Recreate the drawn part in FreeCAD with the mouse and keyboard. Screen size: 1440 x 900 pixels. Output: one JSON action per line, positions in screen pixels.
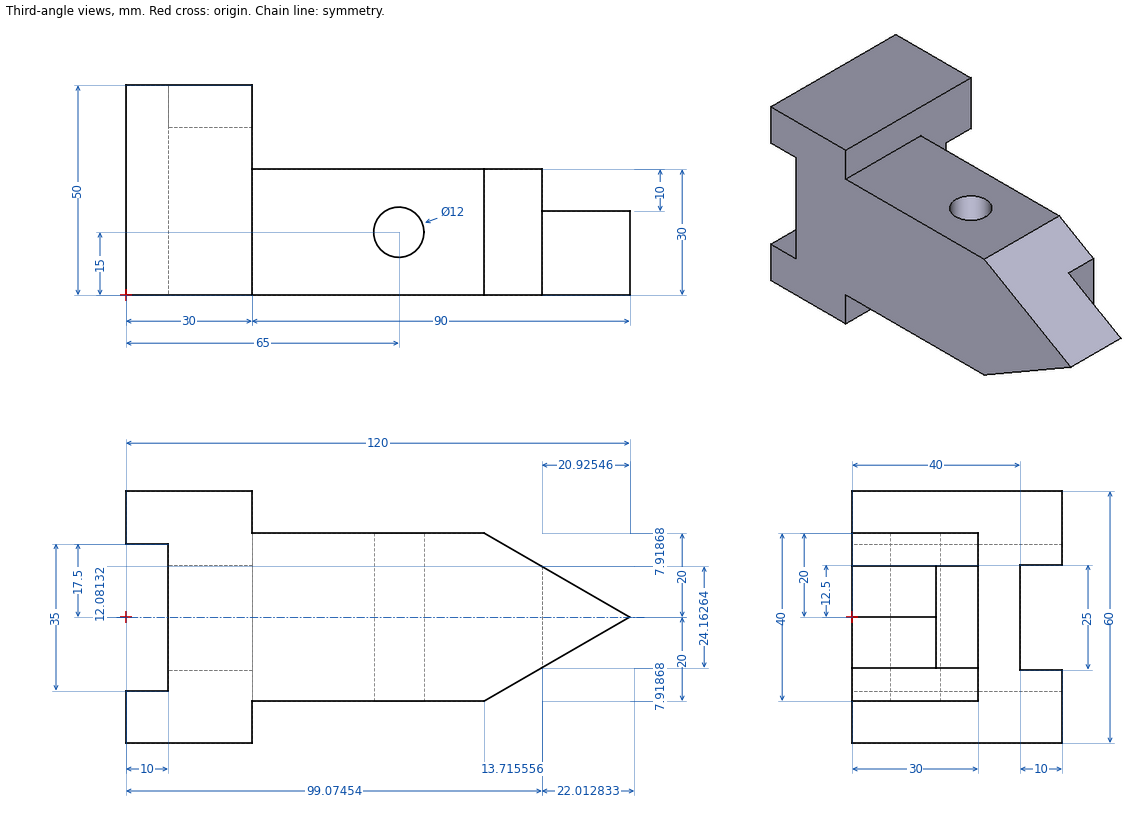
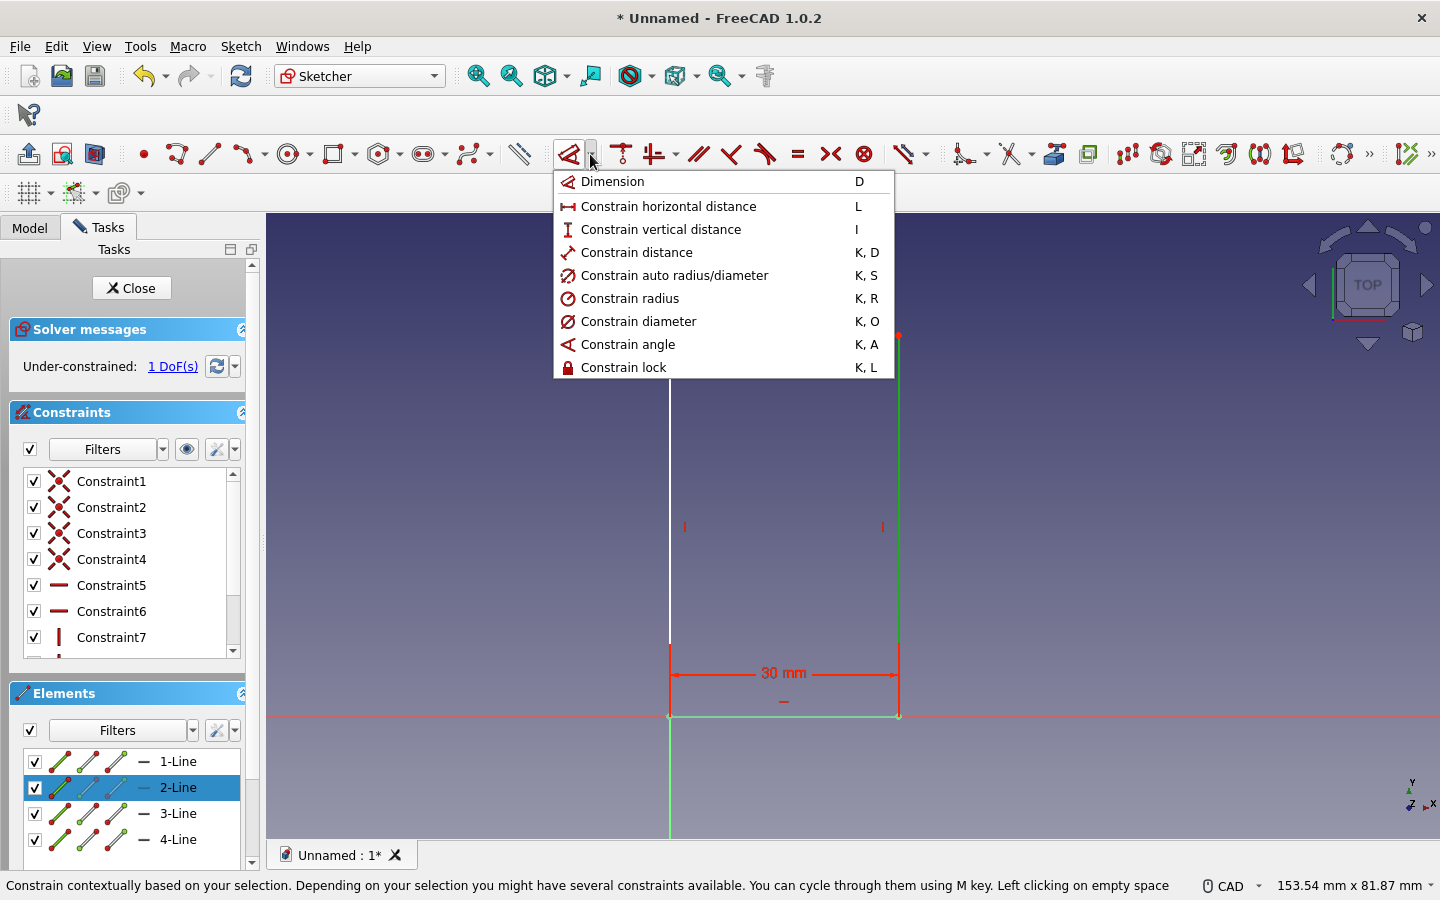
{"action": "left_click", "coordinate": [724, 230]}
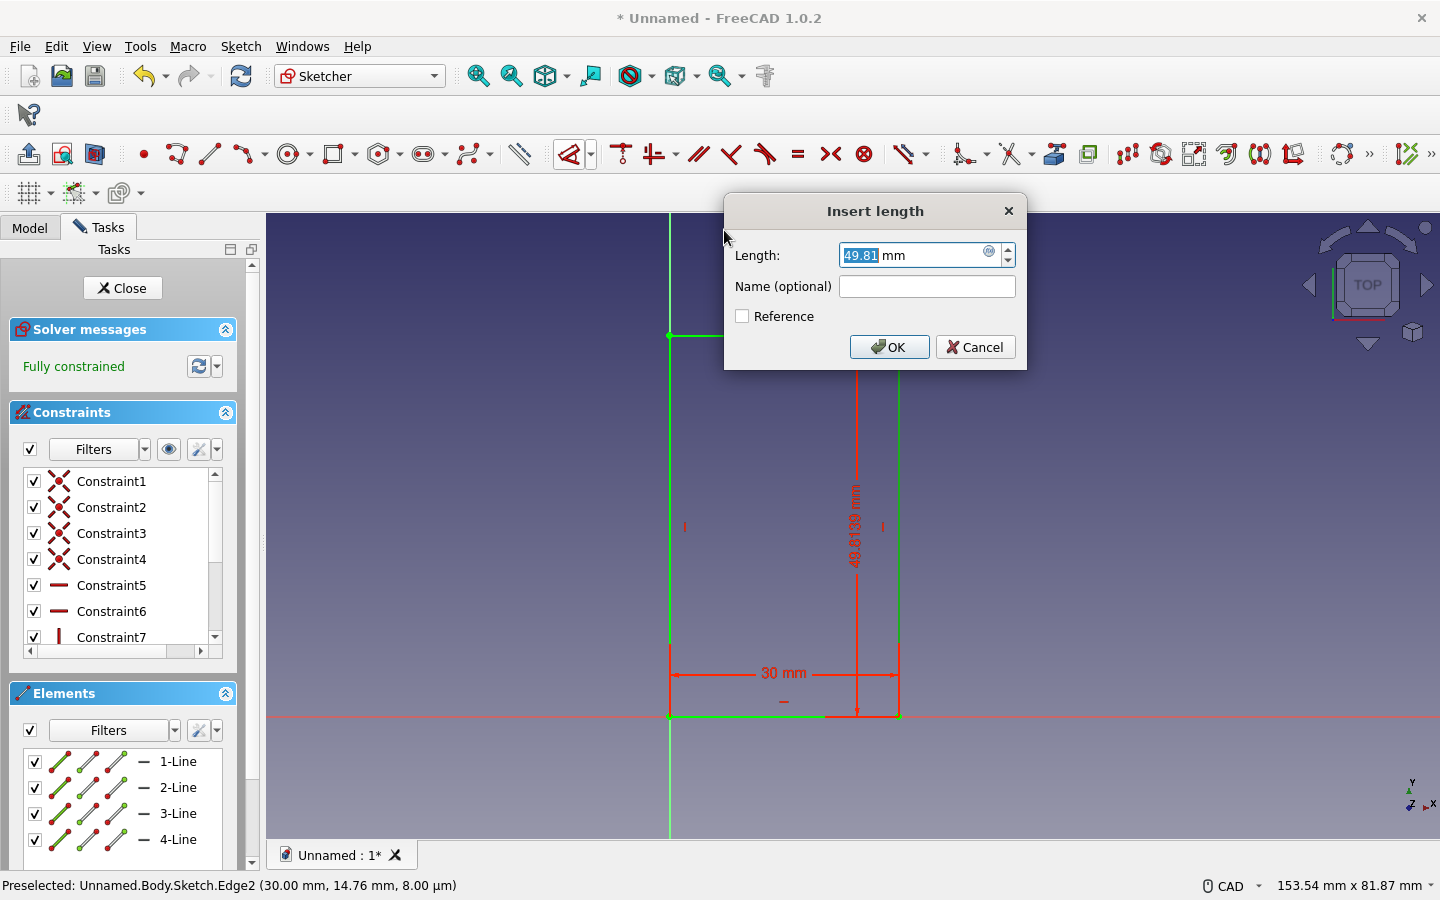
{"action": "type", "text": "50"}
{"action": "key", "text": "Return"}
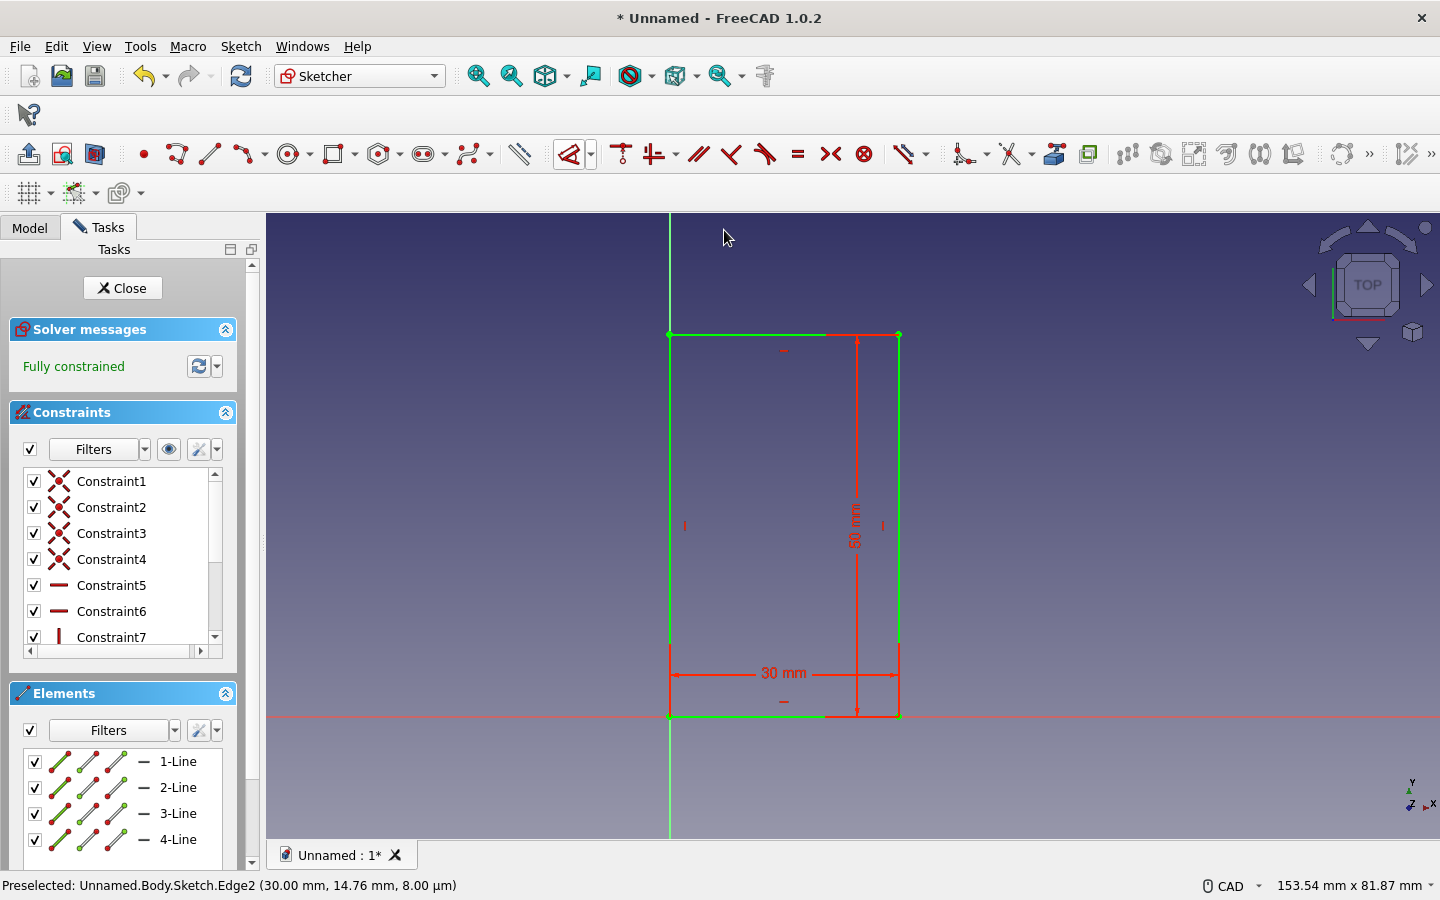
{"action": "left_click", "coordinate": [123, 288]}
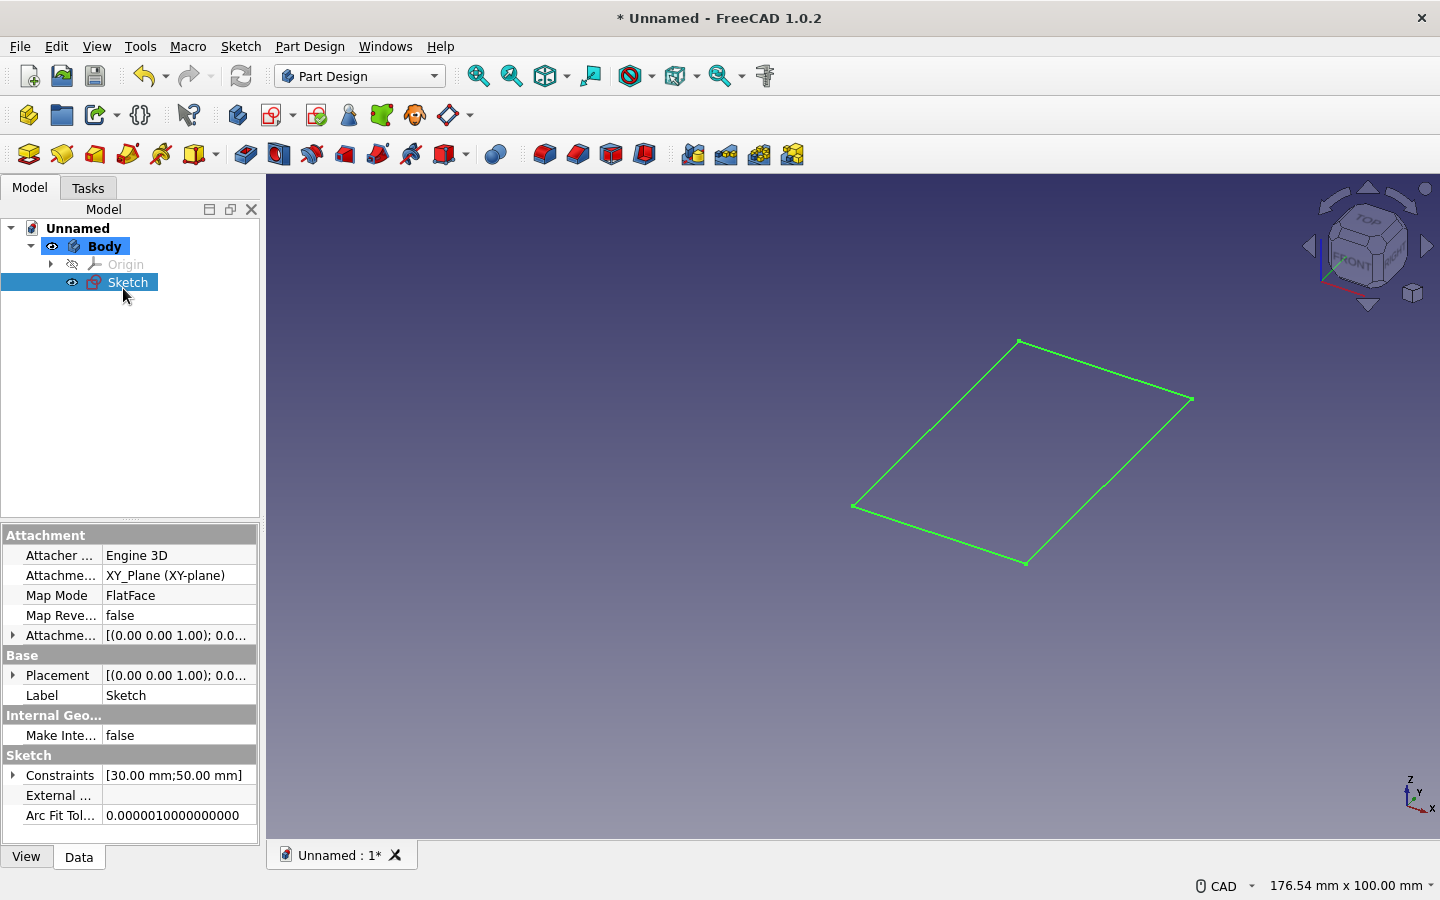
{"action": "left_click", "coordinate": [29, 154]}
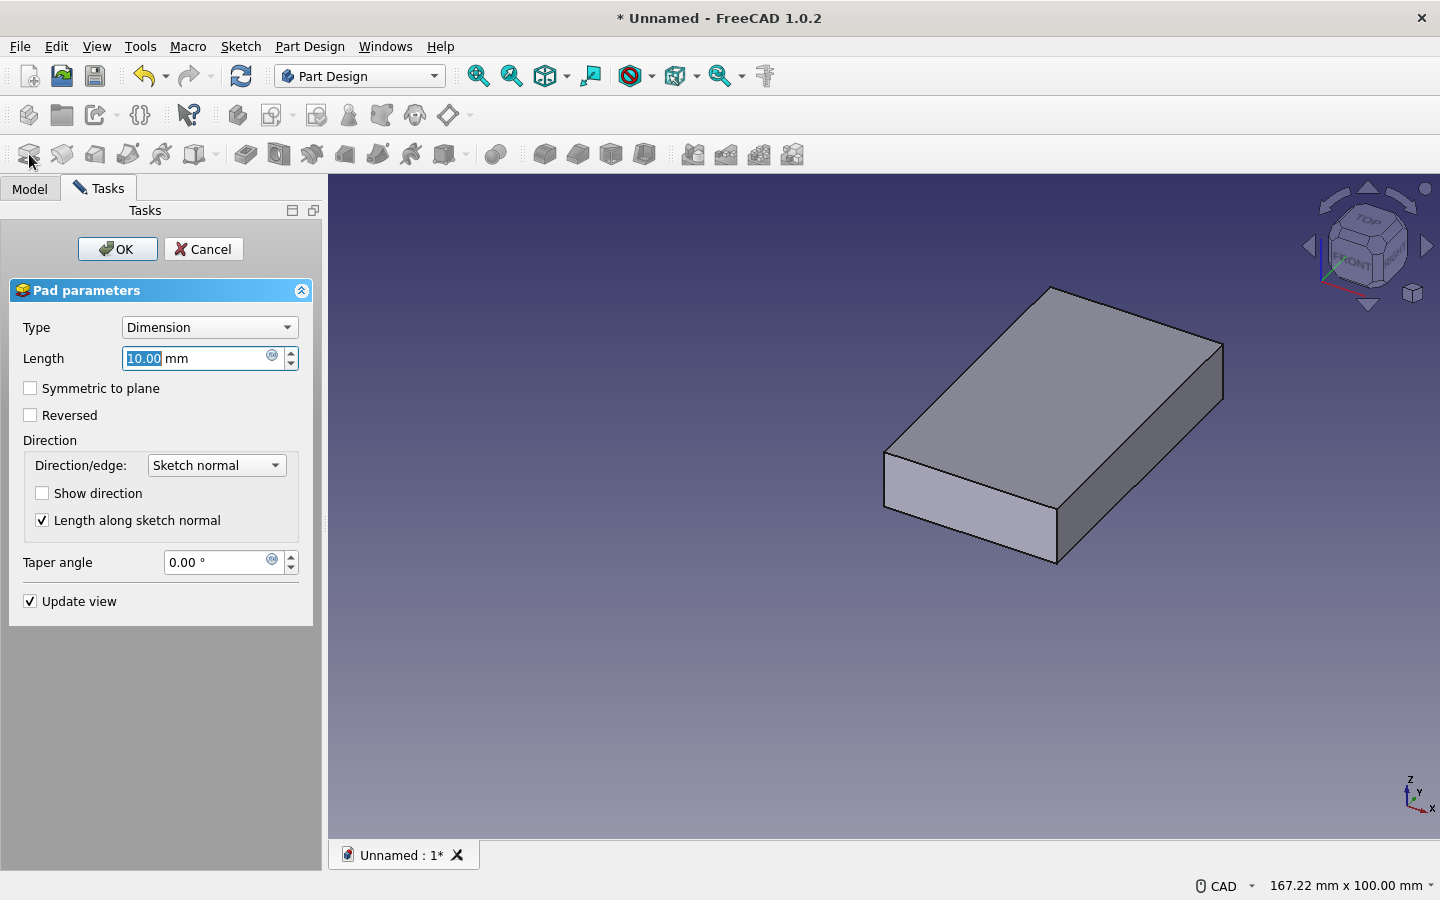
{"action": "type", "text": "60"}
{"action": "key", "text": "Tab"}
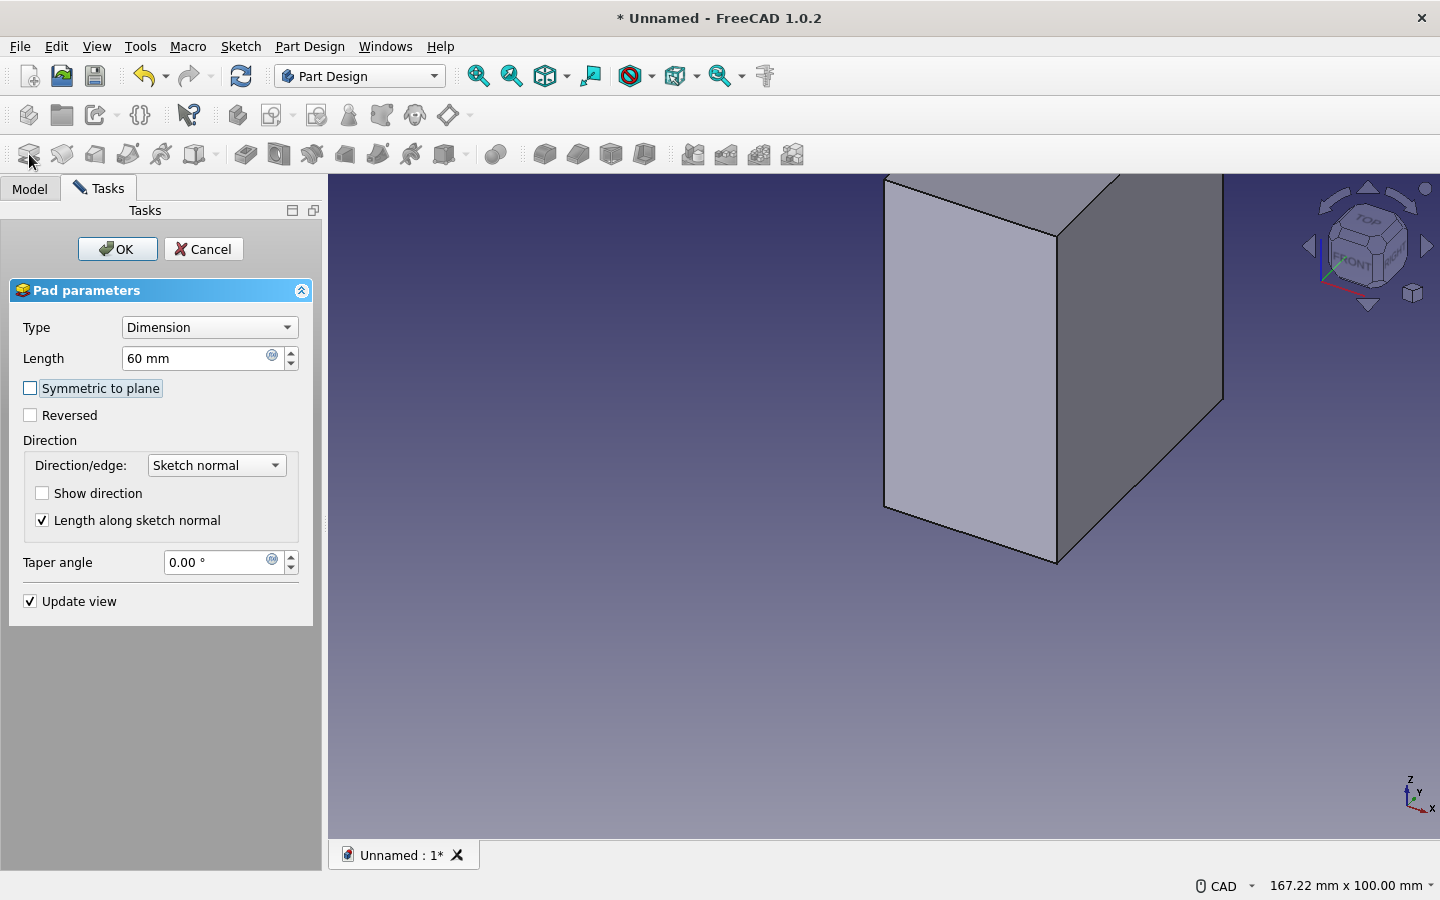
{"action": "left_click", "coordinate": [31, 388]}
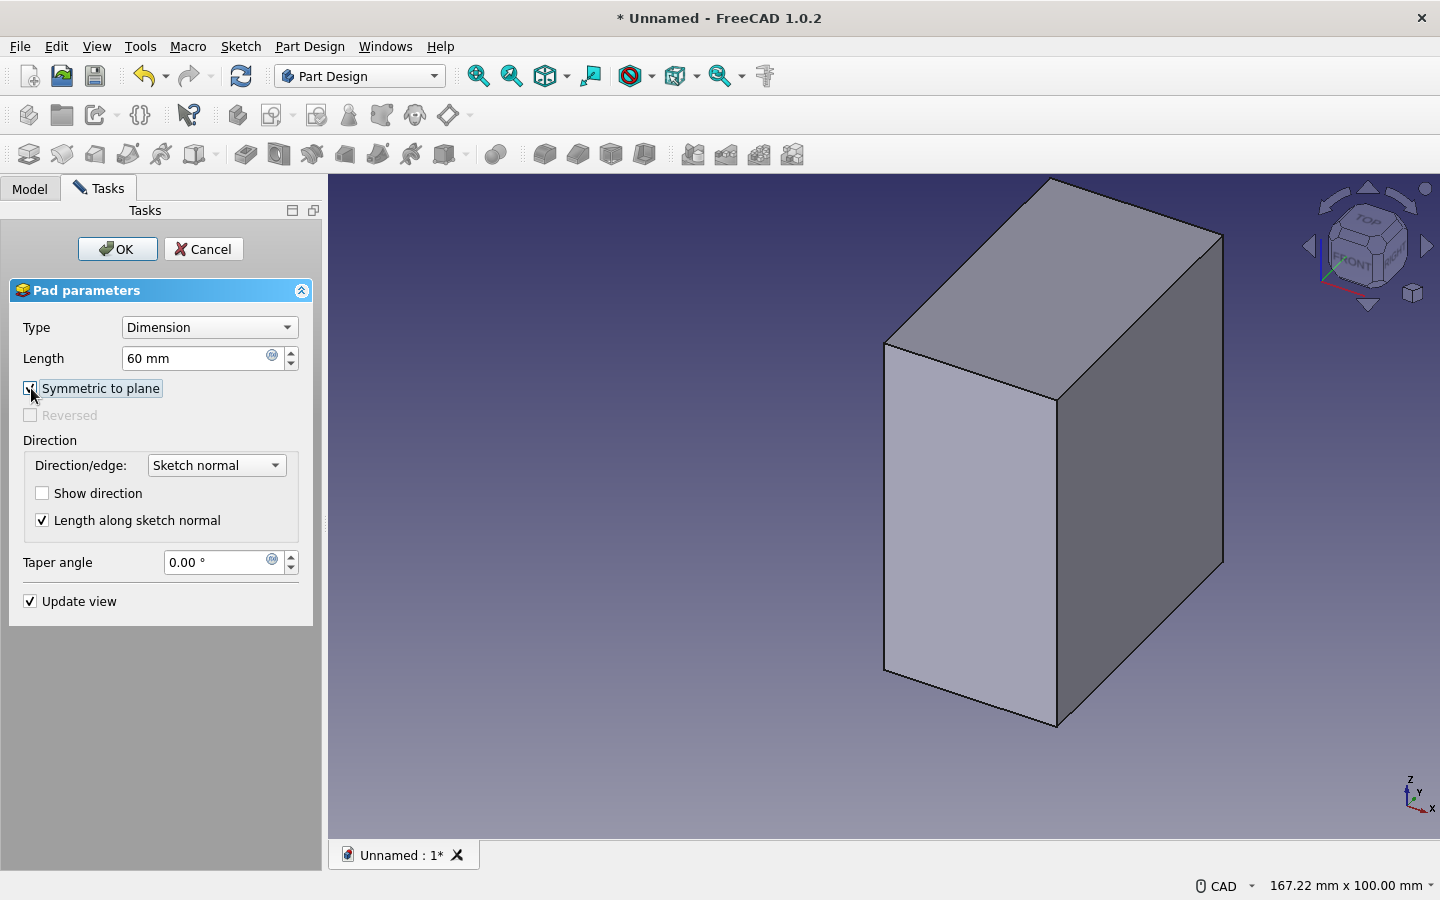
{"action": "left_click", "coordinate": [118, 249]}